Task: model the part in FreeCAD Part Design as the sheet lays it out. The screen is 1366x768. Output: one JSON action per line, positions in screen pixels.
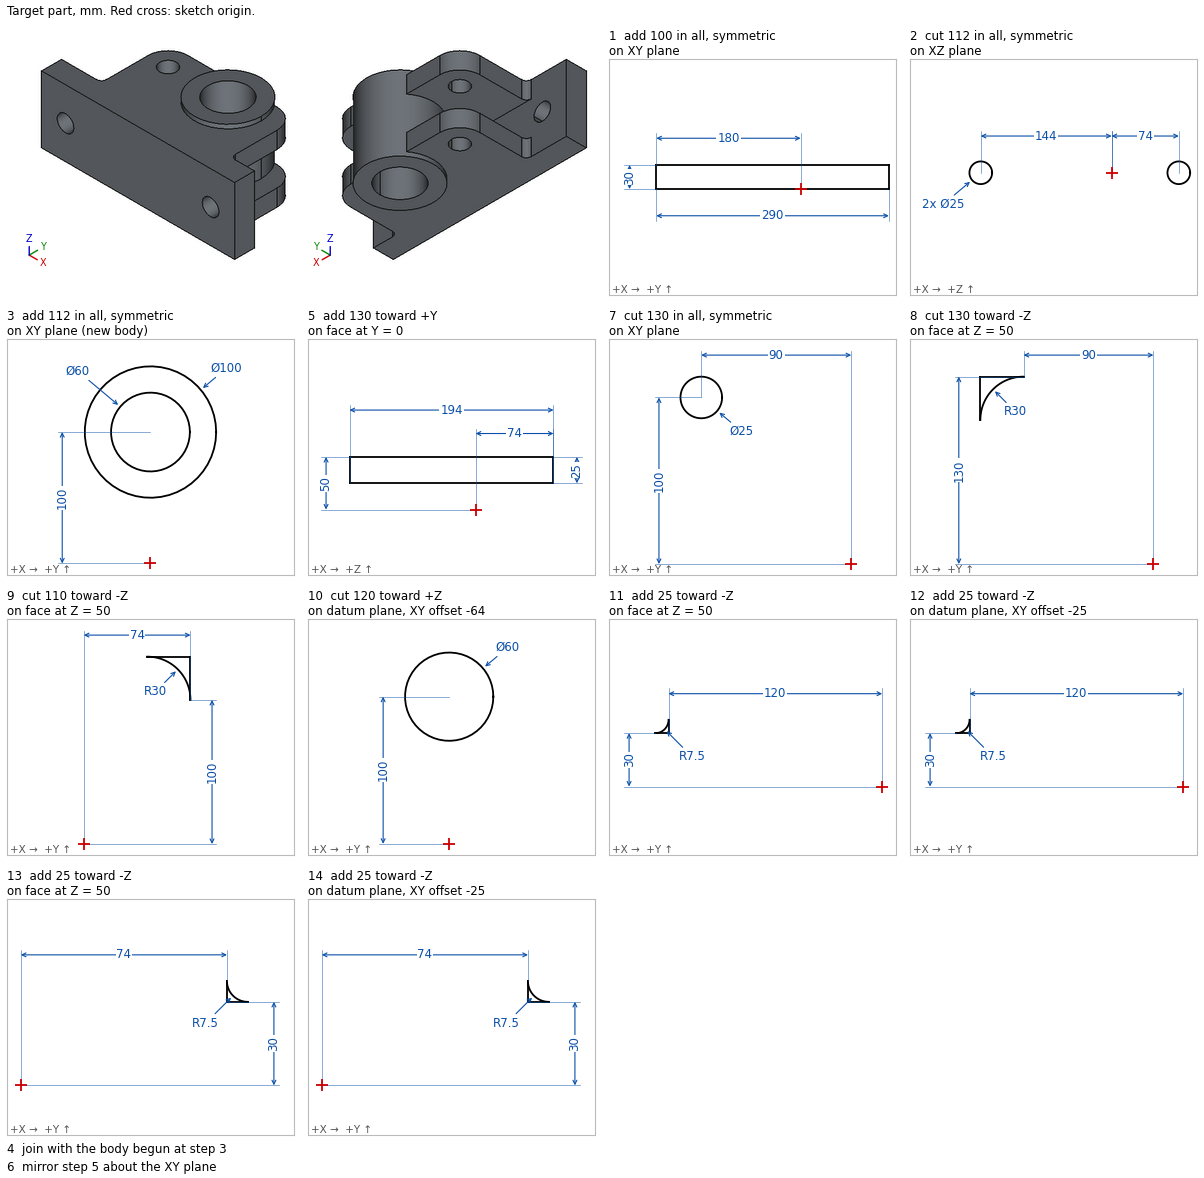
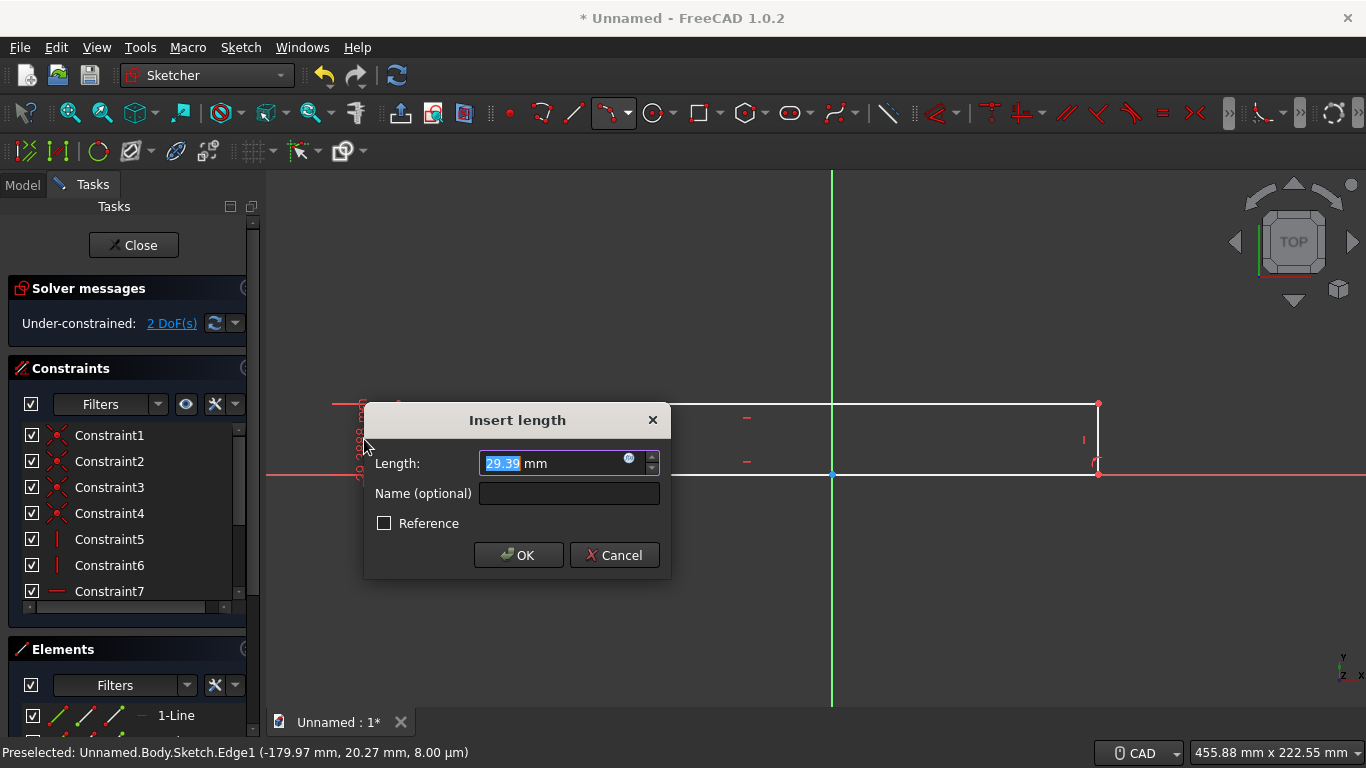
{"action": "type", "text": "30"}
{"action": "key", "text": "Return"}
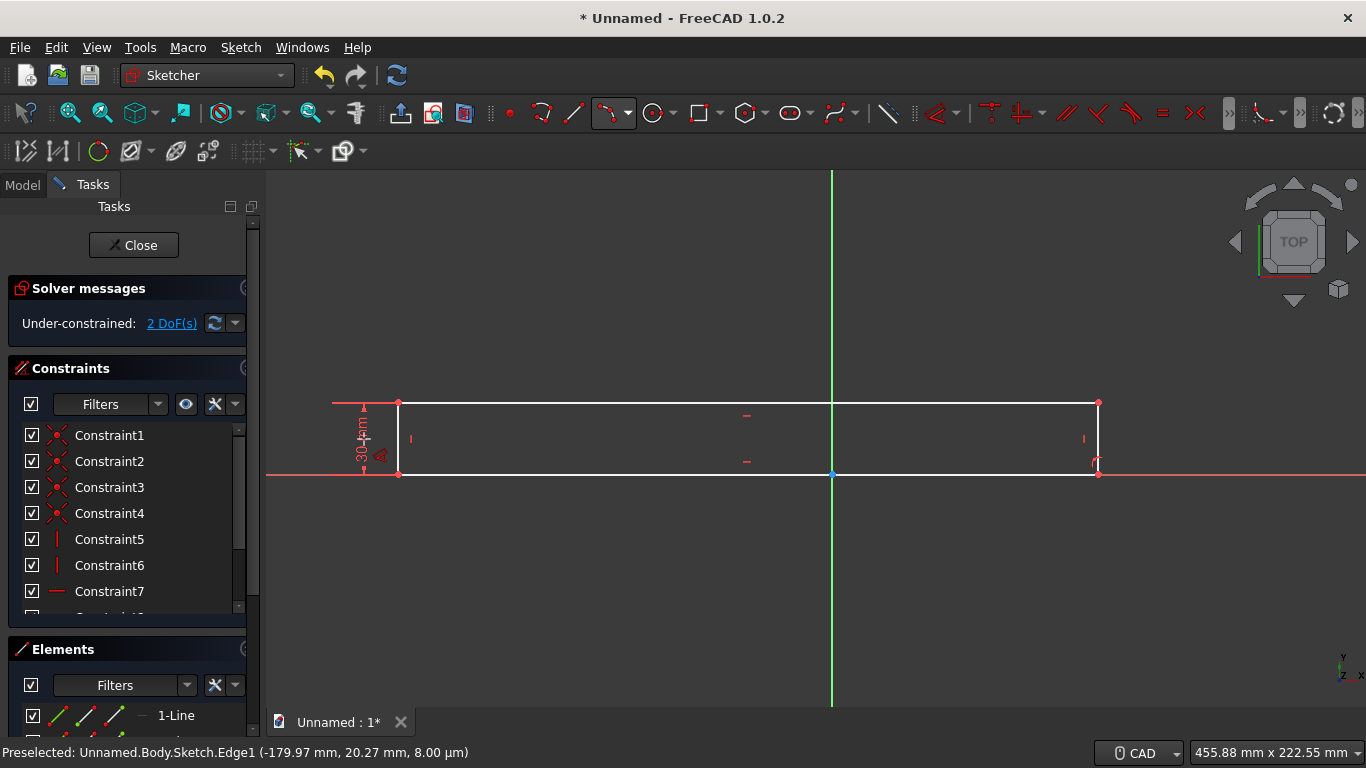
{"action": "left_click", "coordinate": [608, 475]}
{"action": "left_click", "coordinate": [748, 509]}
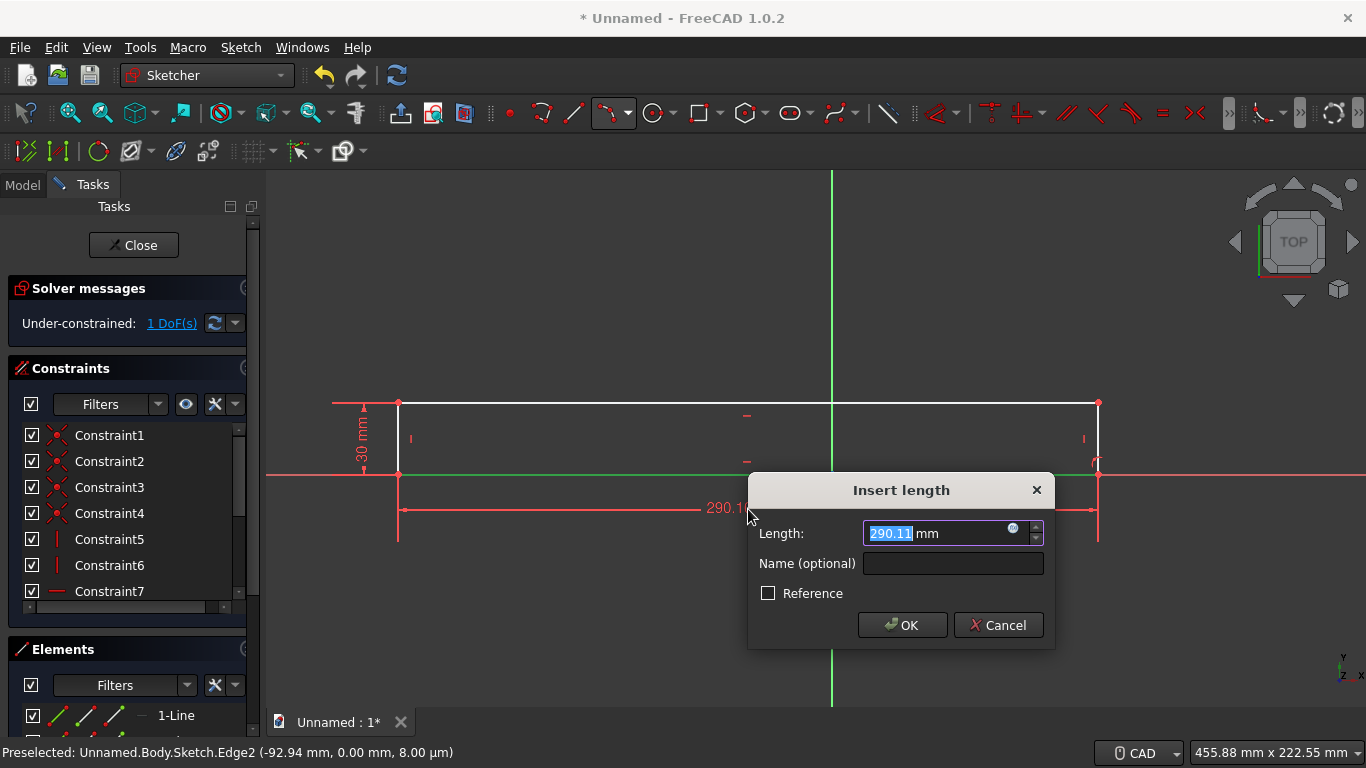
{"action": "type", "text": "290"}
{"action": "key", "text": "Return"}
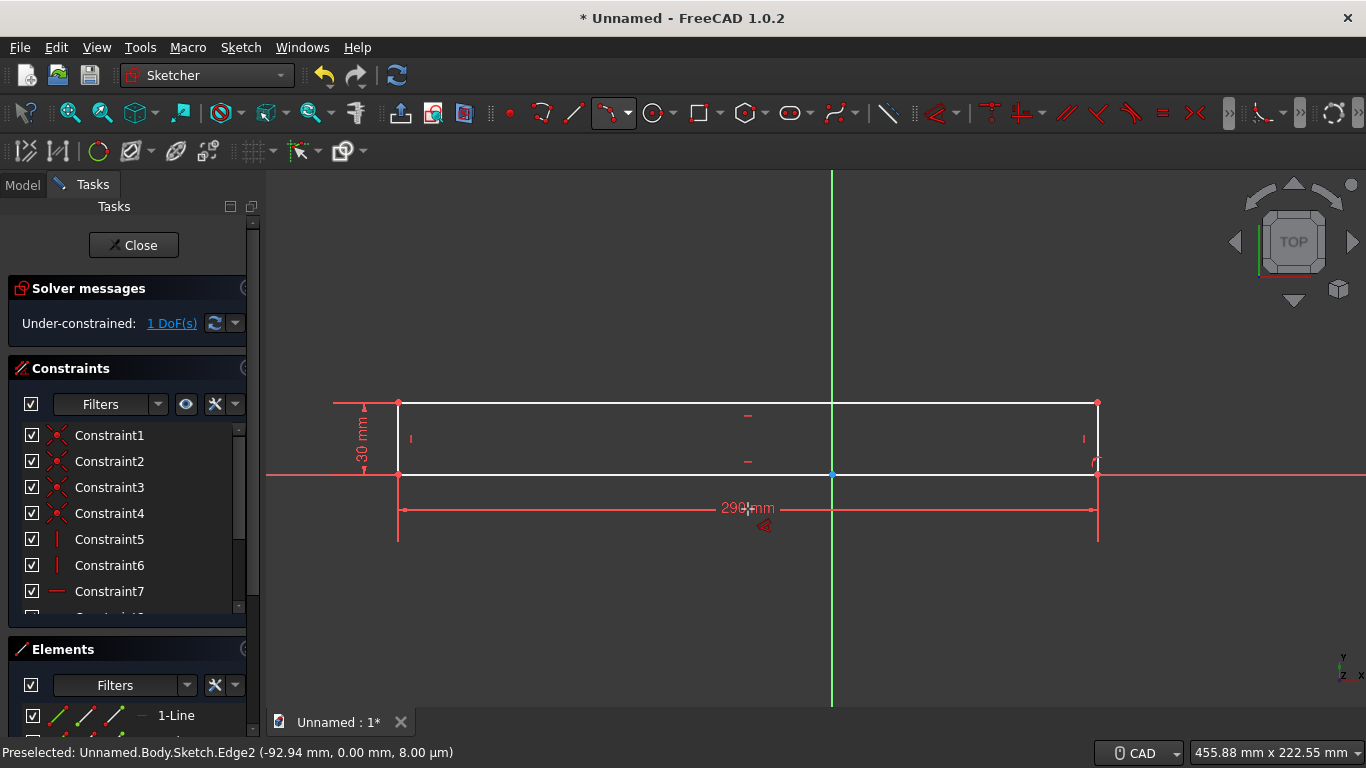
{"action": "left_click", "coordinate": [398, 403]}
{"action": "left_click", "coordinate": [615, 509]}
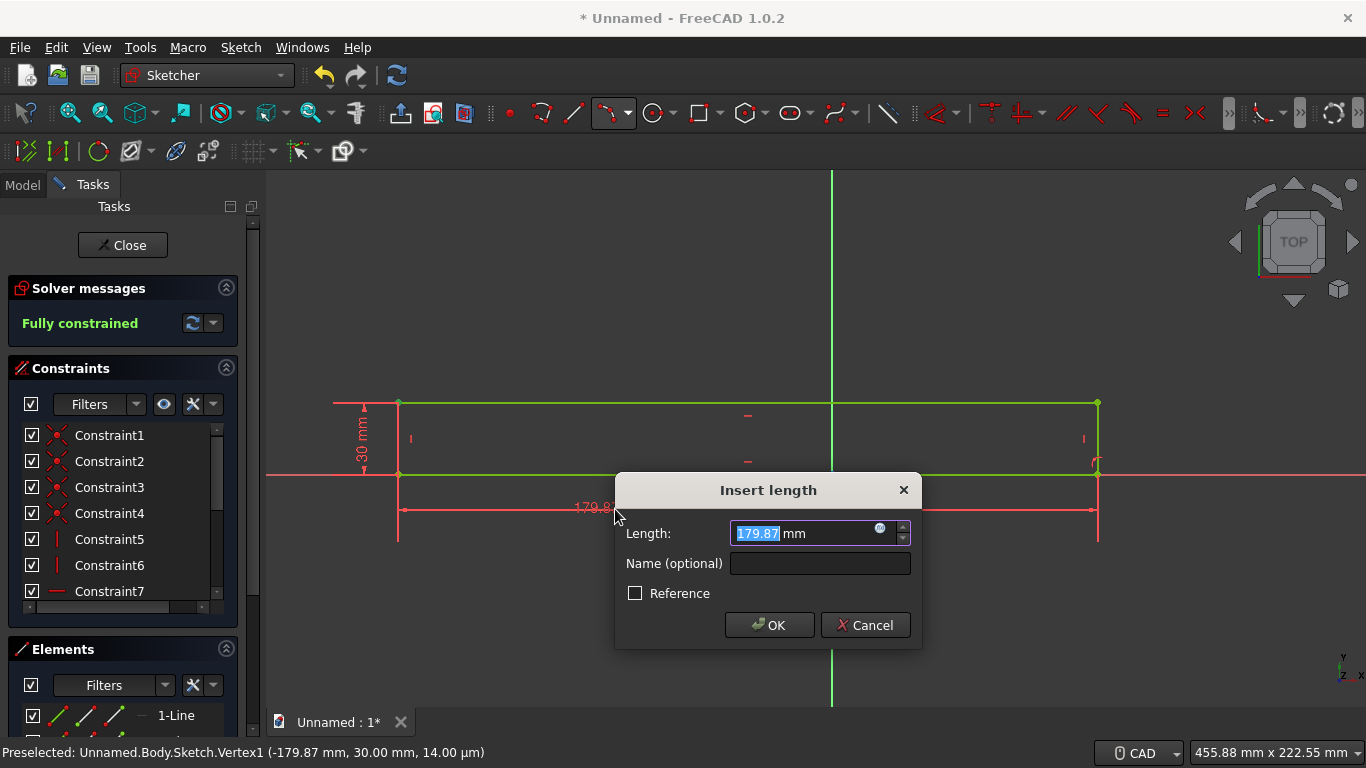
{"action": "type", "text": "180"}
{"action": "key", "text": "Return"}
{"action": "key", "text": "Escape"}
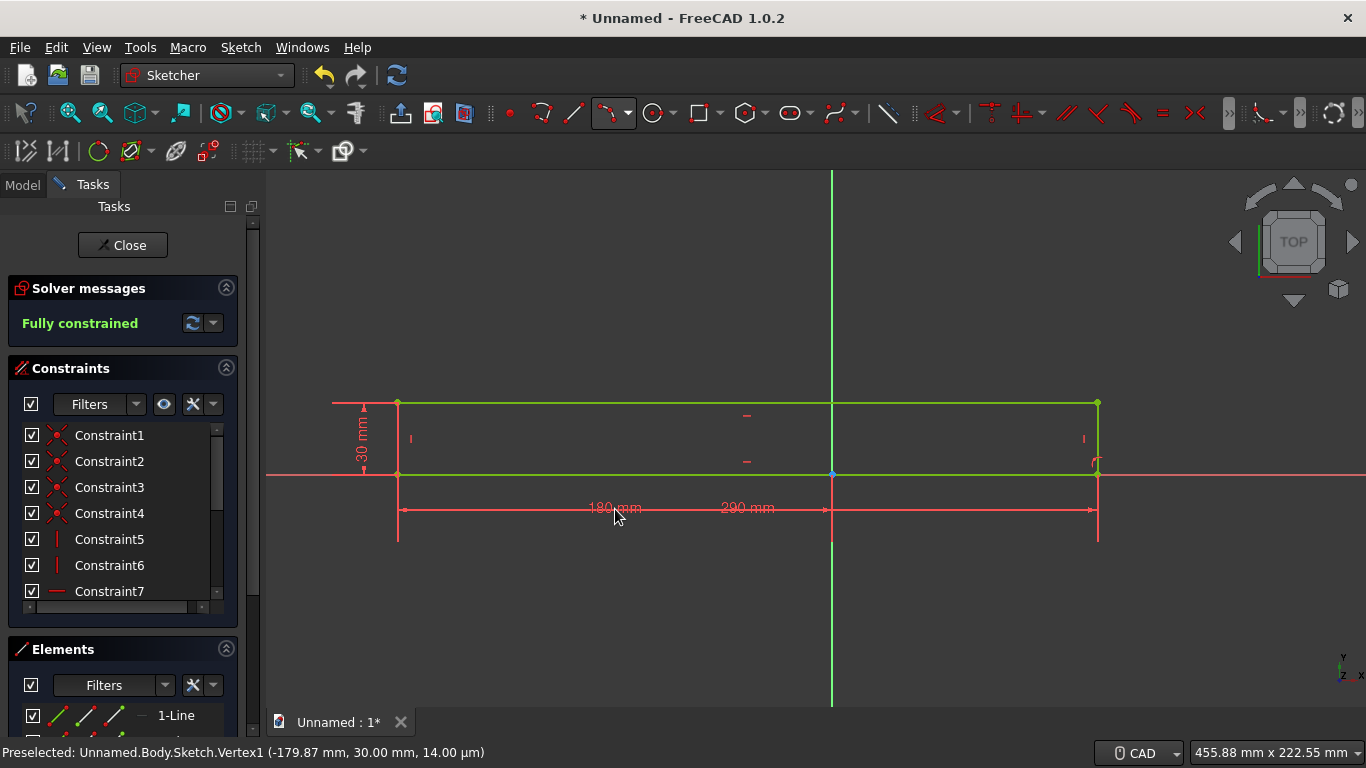
{"action": "left_click", "coordinate": [123, 245]}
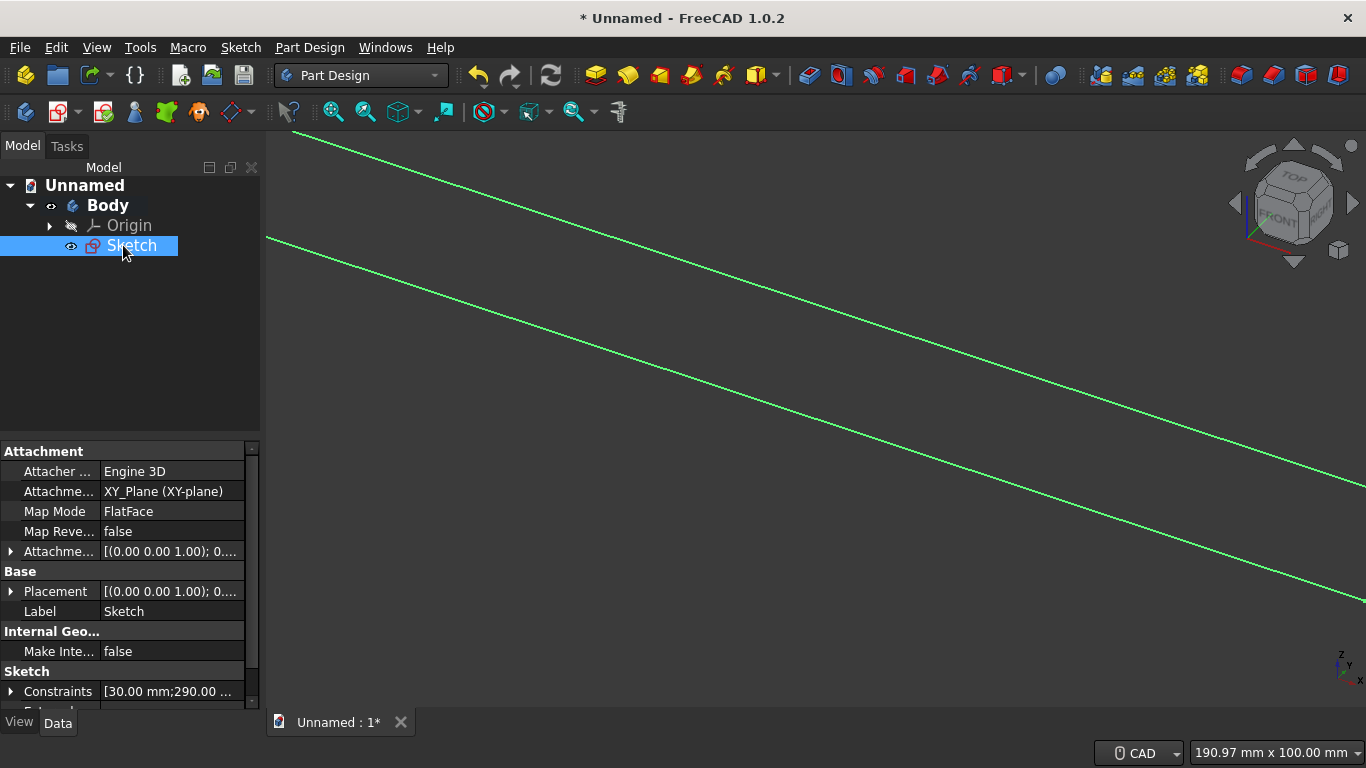
{"action": "left_click", "coordinate": [596, 76]}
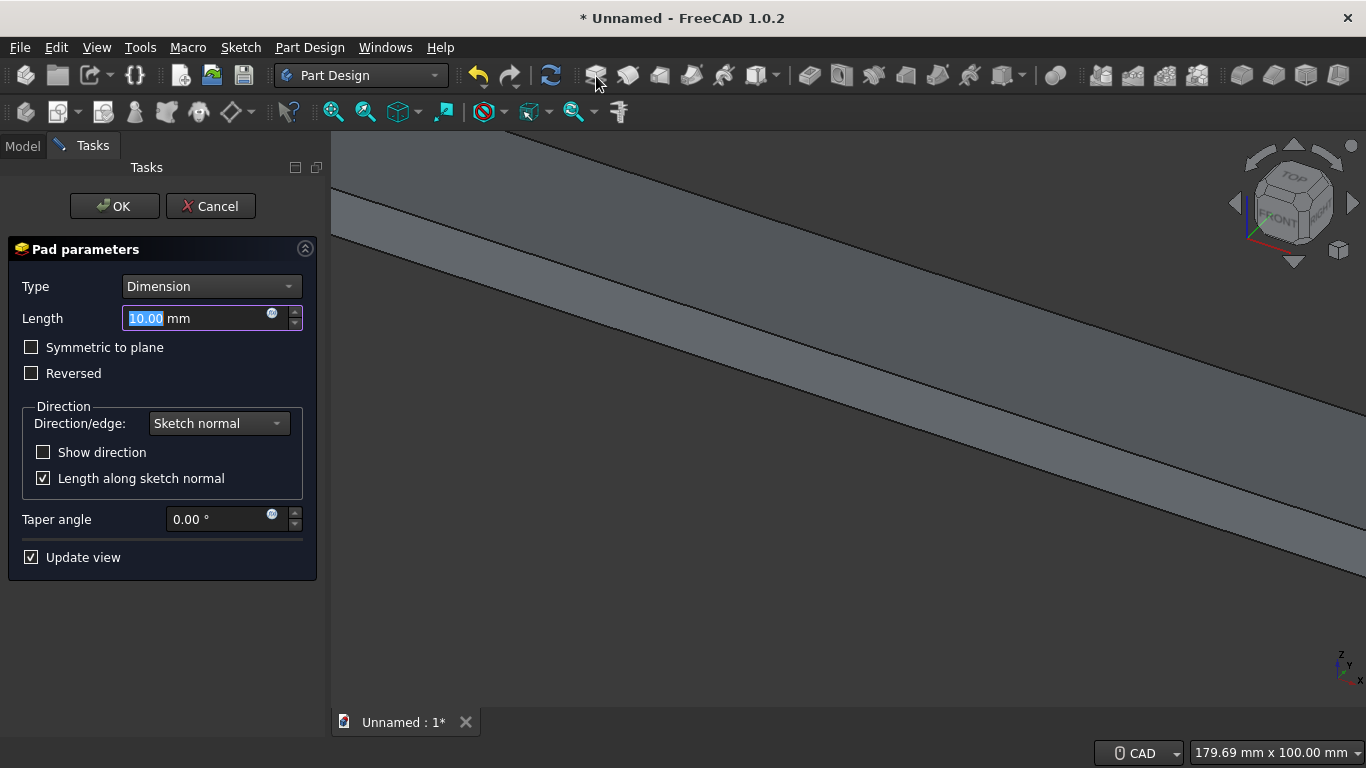
{"action": "type", "text": "100"}
{"action": "key", "text": "Tab"}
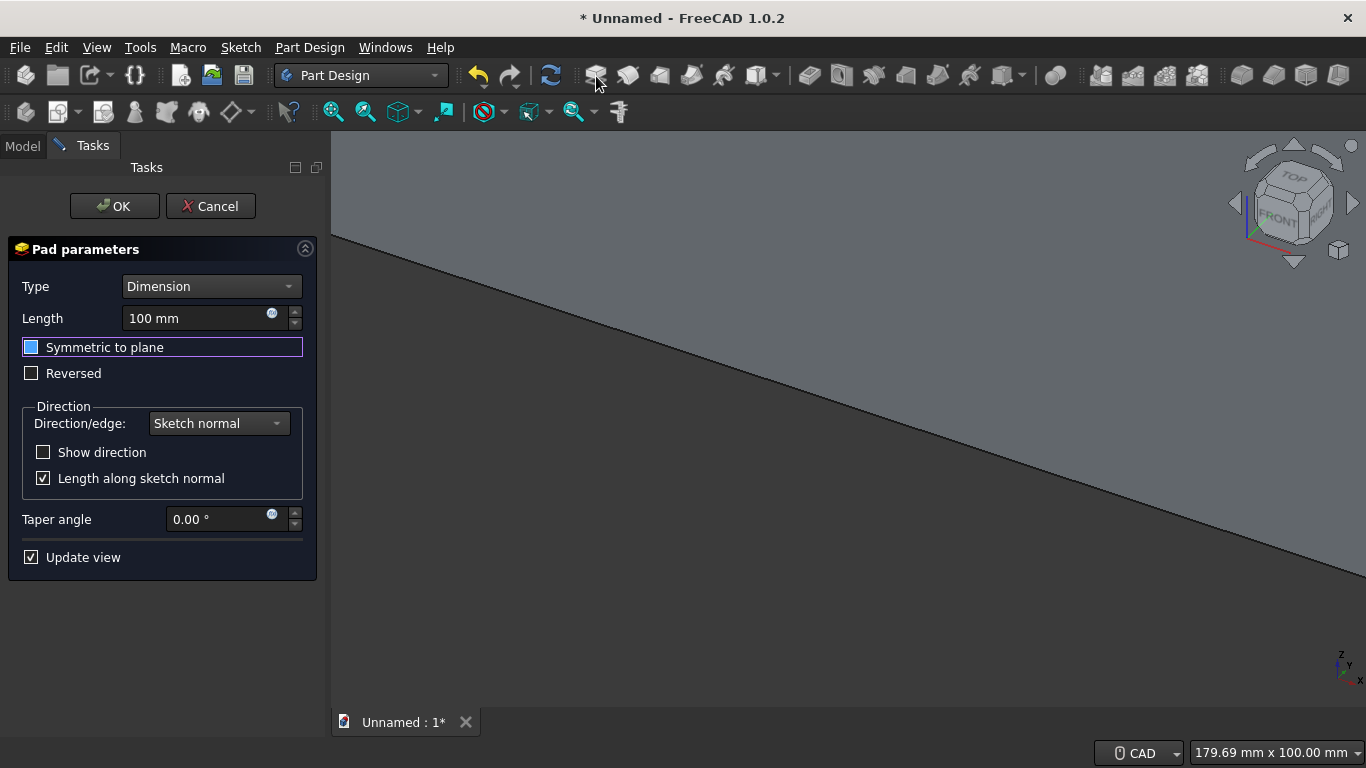
{"action": "left_click", "coordinate": [30, 347]}